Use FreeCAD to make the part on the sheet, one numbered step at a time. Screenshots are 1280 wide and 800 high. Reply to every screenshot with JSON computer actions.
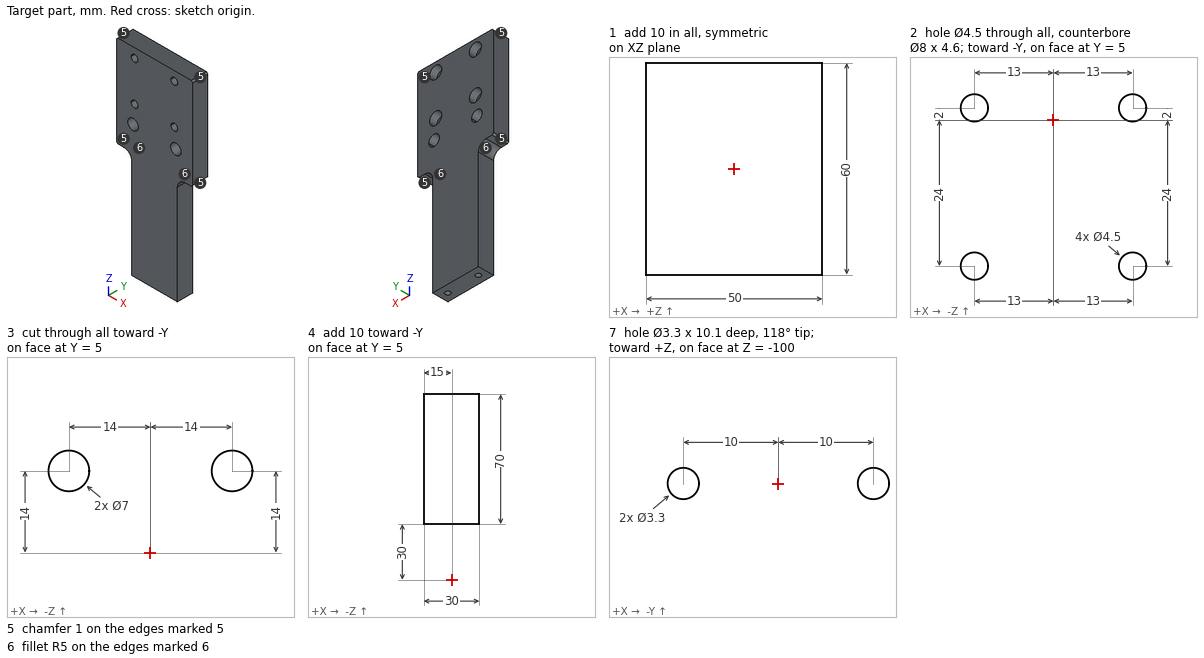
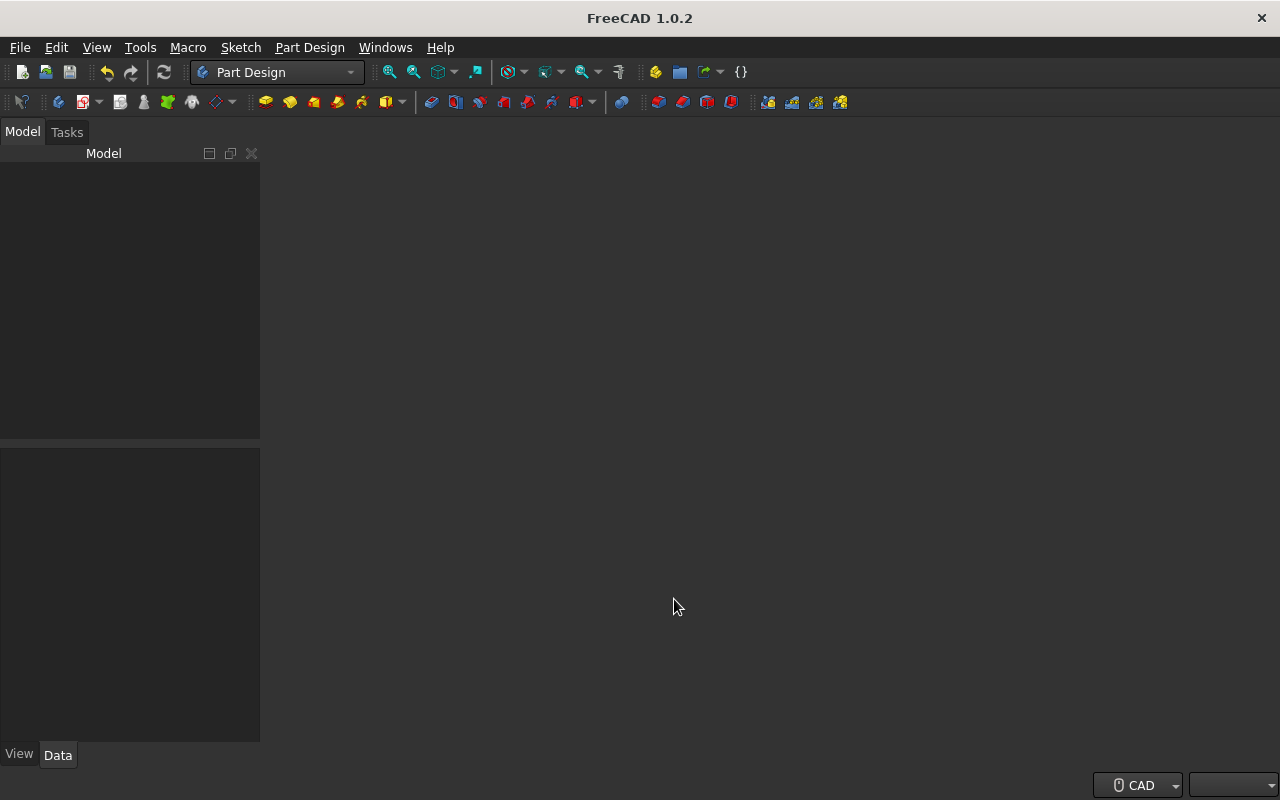
{"action": "left_click", "coordinate": [22, 72]}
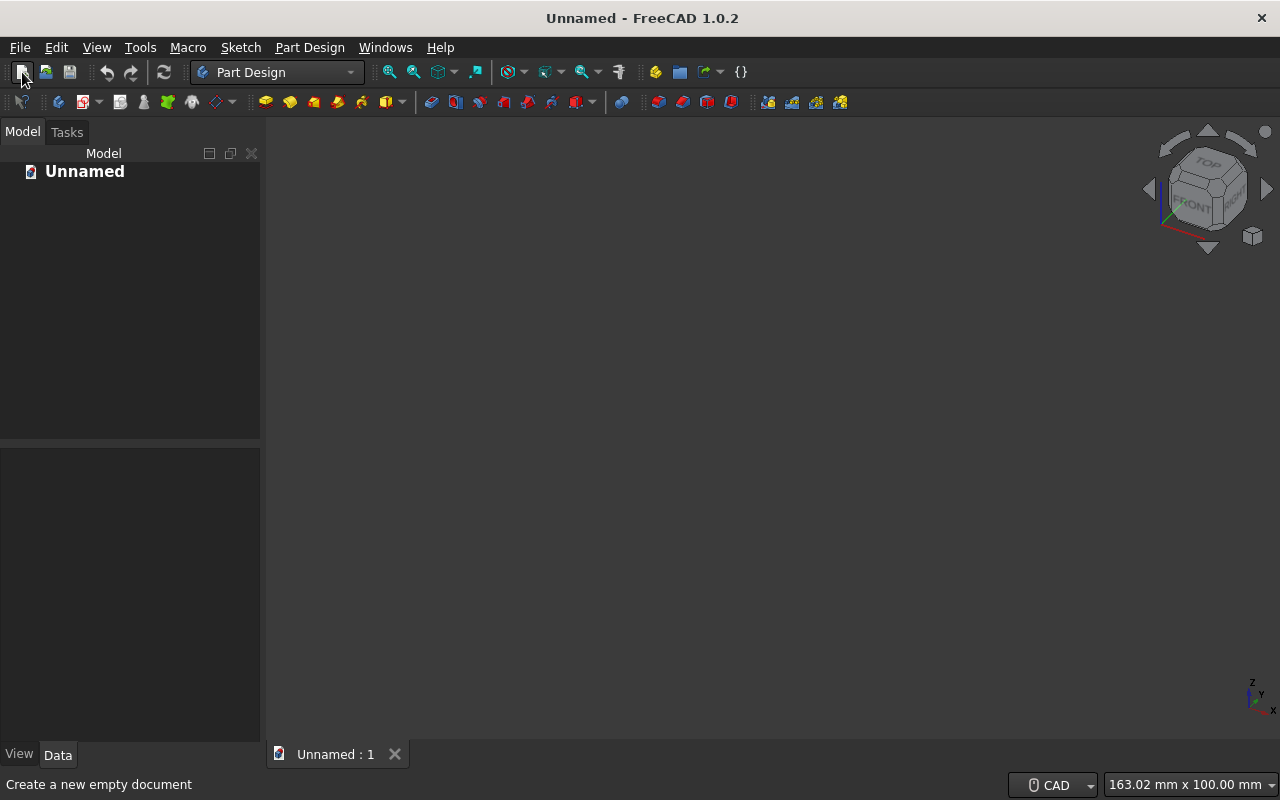
{"action": "left_click", "coordinate": [84, 102]}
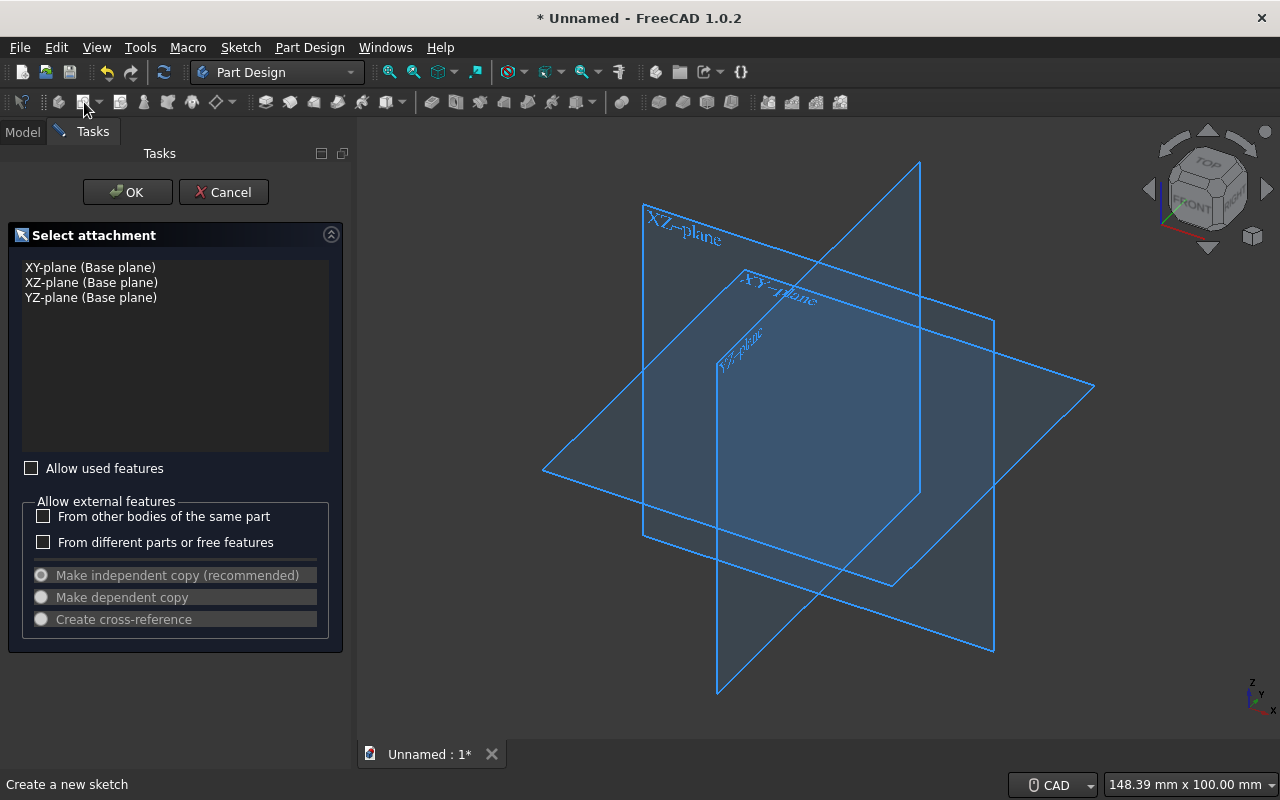
{"action": "left_click", "coordinate": [82, 282]}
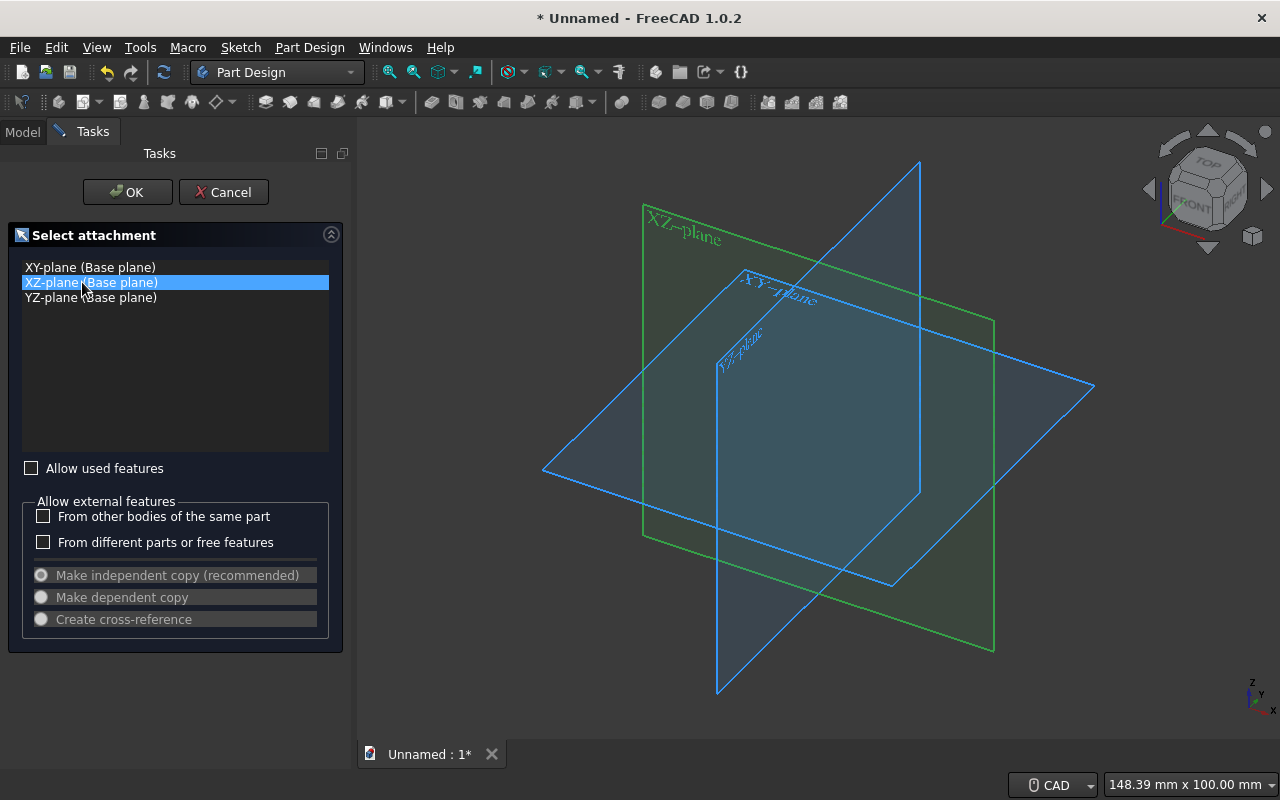
{"action": "left_click", "coordinate": [128, 192]}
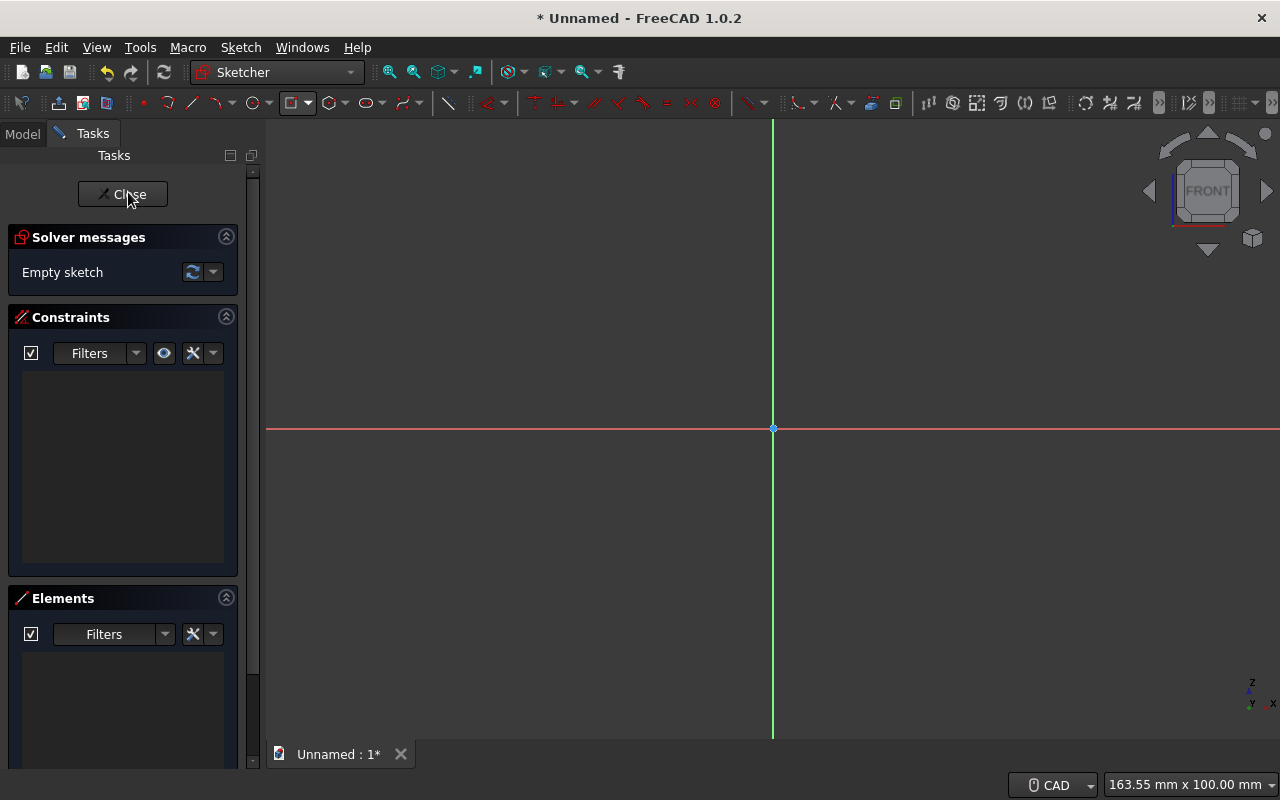
{"action": "left_click", "coordinate": [292, 104]}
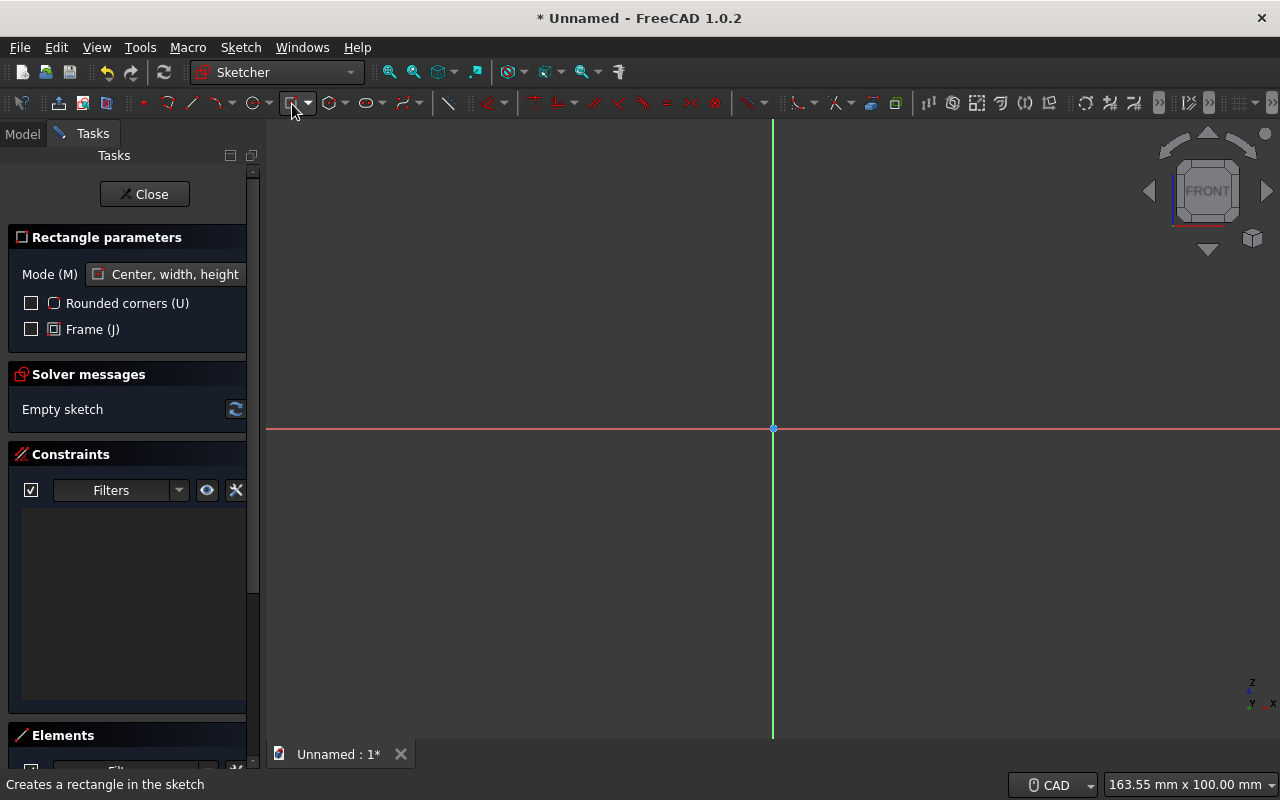
{"action": "left_click", "coordinate": [773, 429]}
{"action": "mouse_move", "coordinate": [928, 243]}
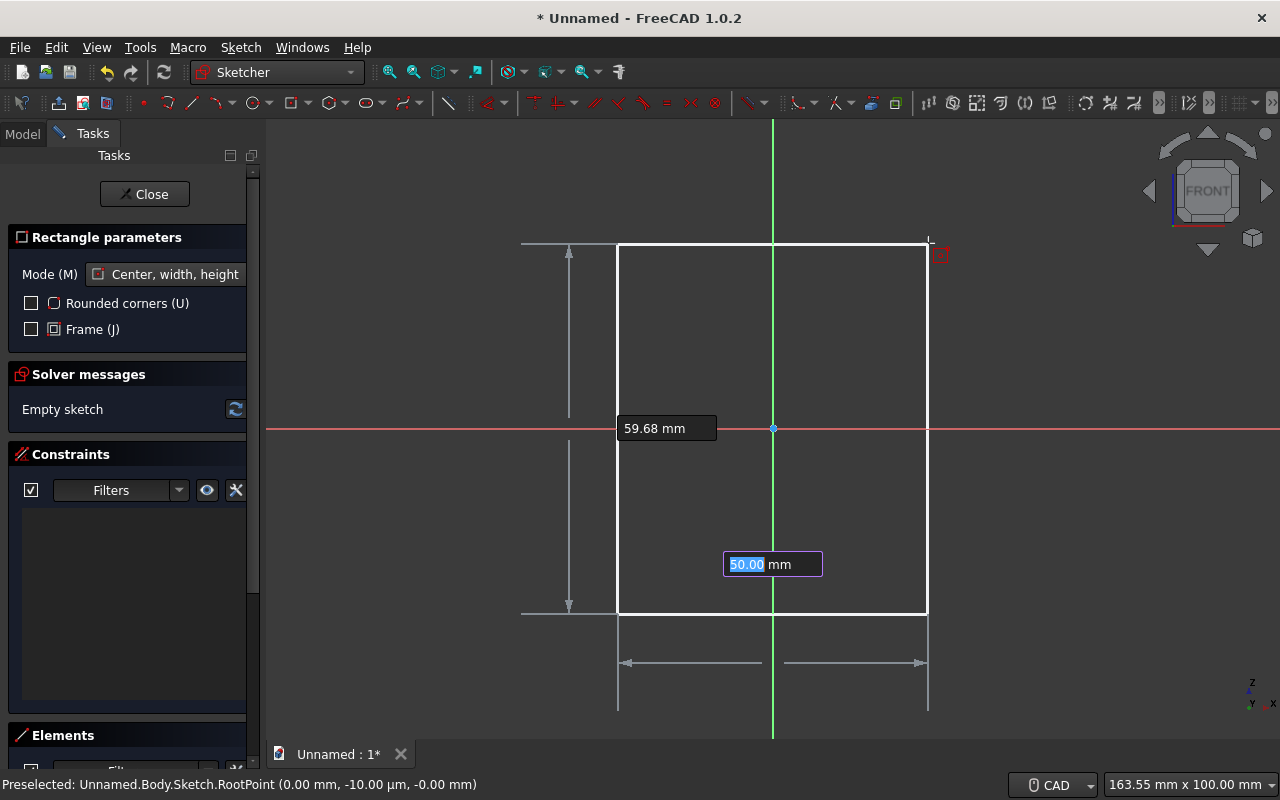
{"action": "type", "text": "50"}
{"action": "key", "text": "Tab"}
{"action": "type", "text": "60"}
{"action": "key", "text": "Return"}
{"action": "key", "text": "Escape"}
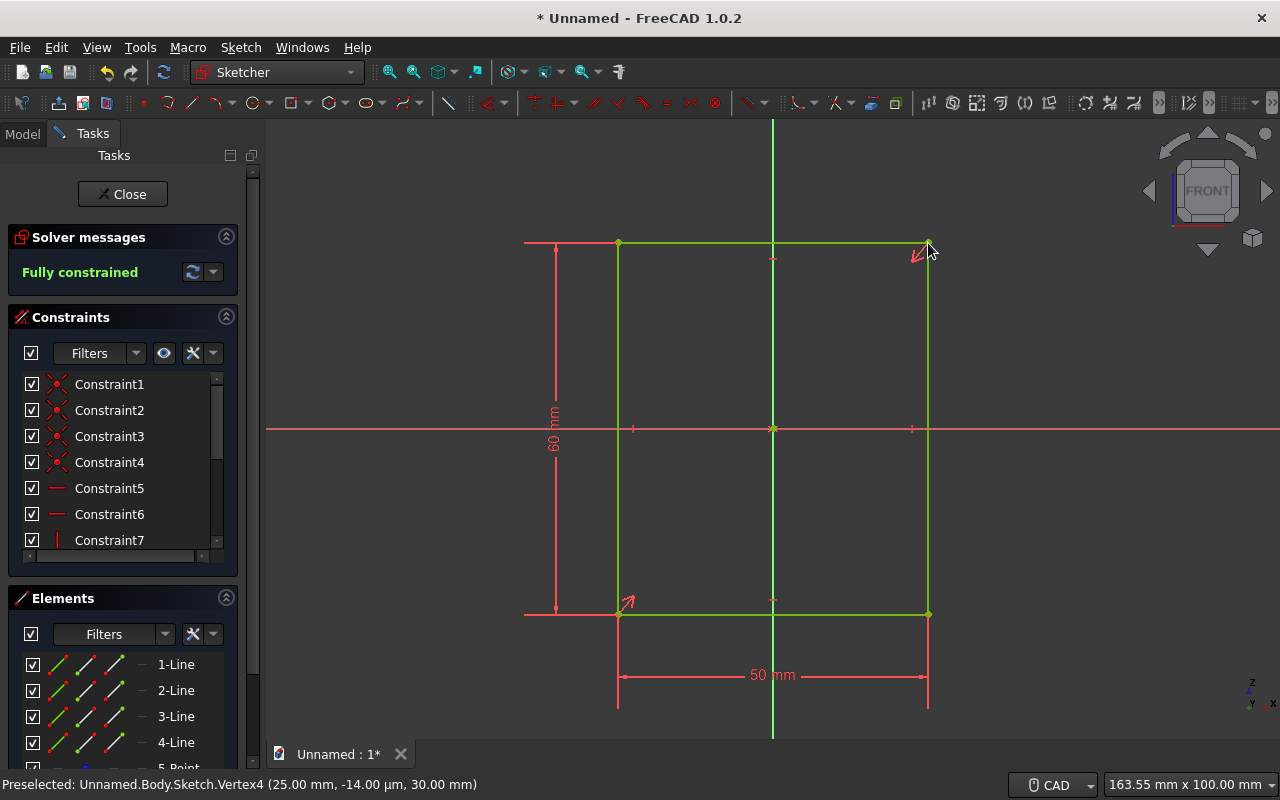
{"action": "left_click", "coordinate": [123, 194]}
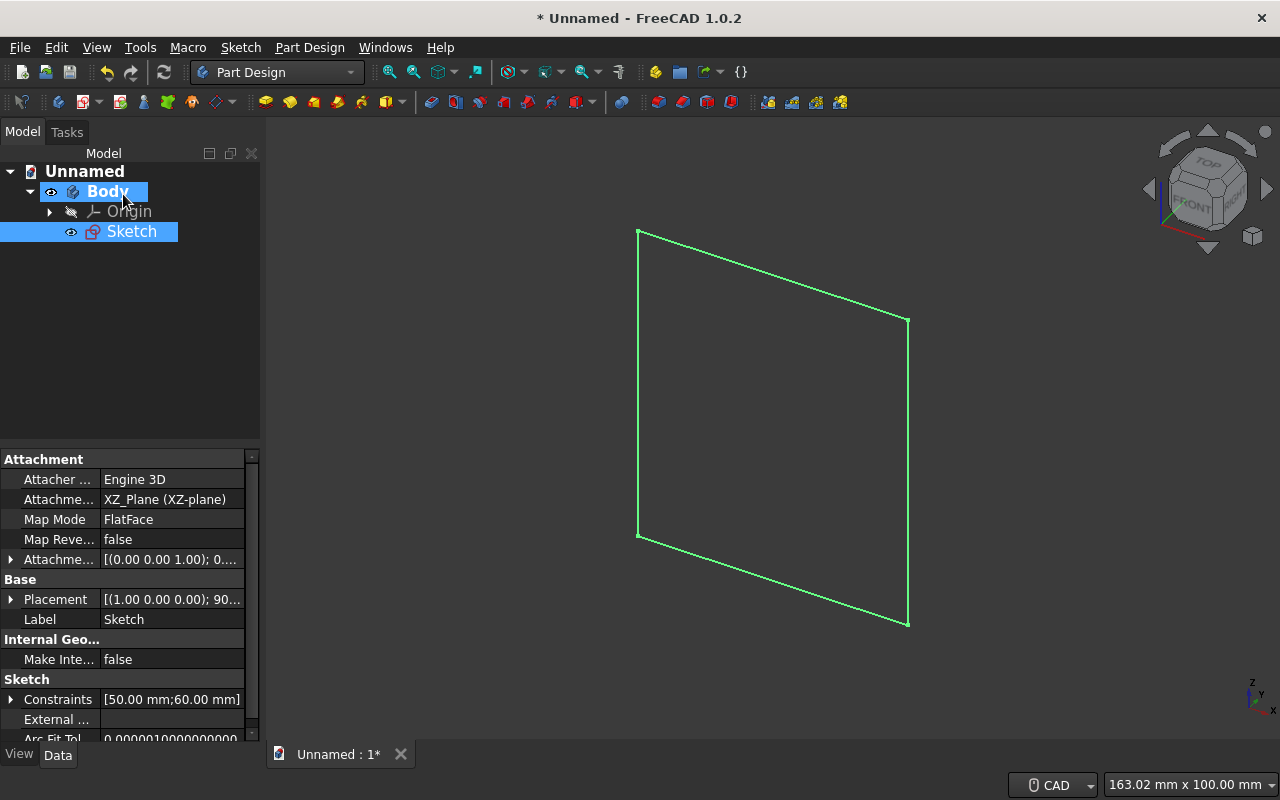
{"action": "left_click", "coordinate": [266, 102]}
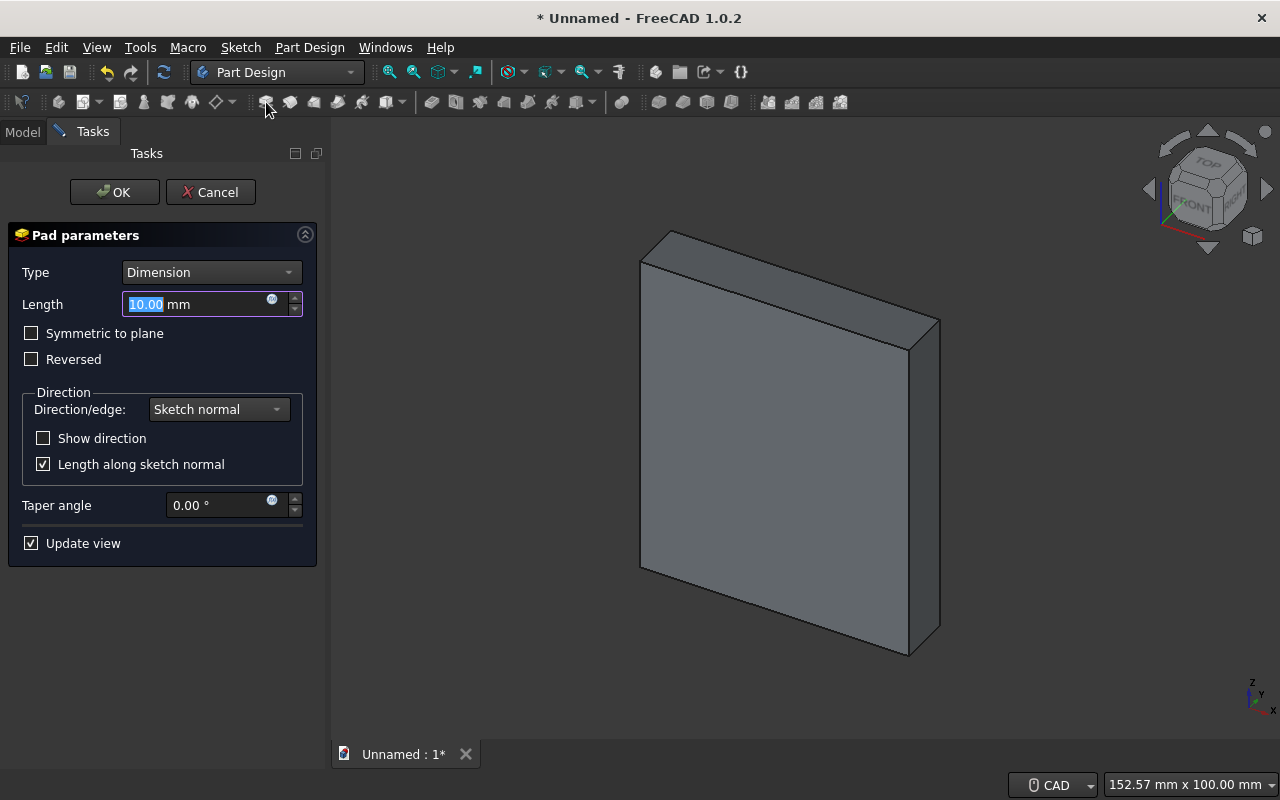
{"action": "type", "text": "10"}
{"action": "key", "text": "Tab"}